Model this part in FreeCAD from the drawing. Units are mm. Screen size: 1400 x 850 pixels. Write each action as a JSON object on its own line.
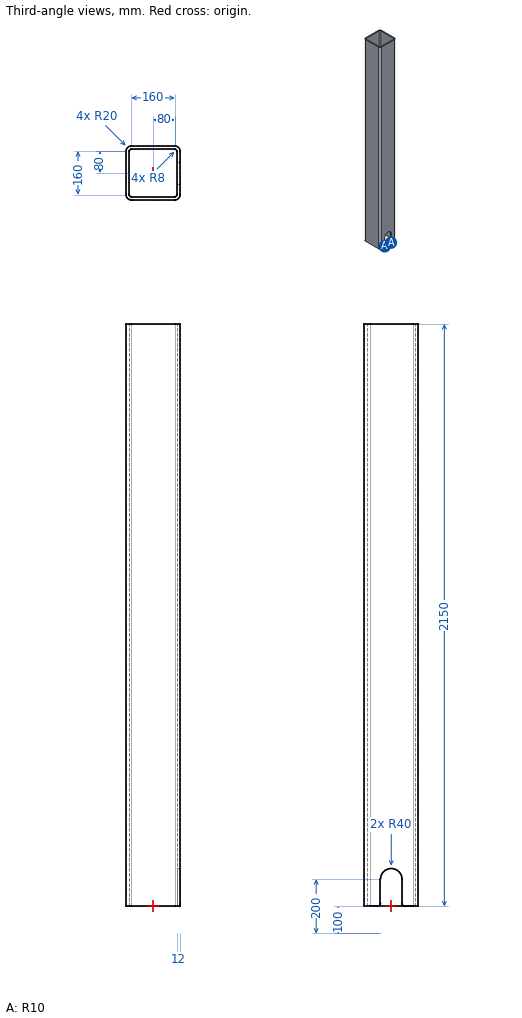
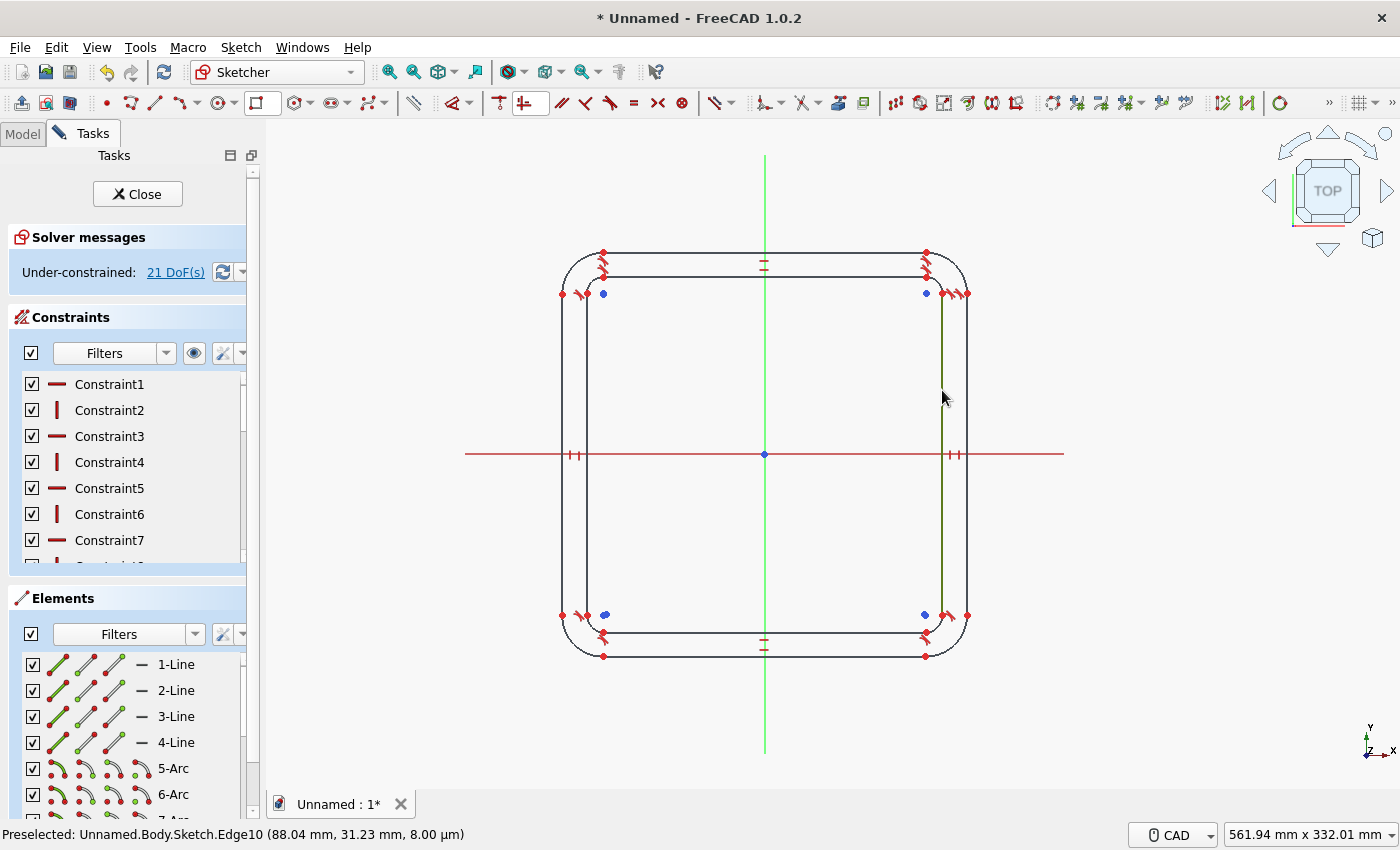
{"action": "left_click", "coordinate": [937, 627]}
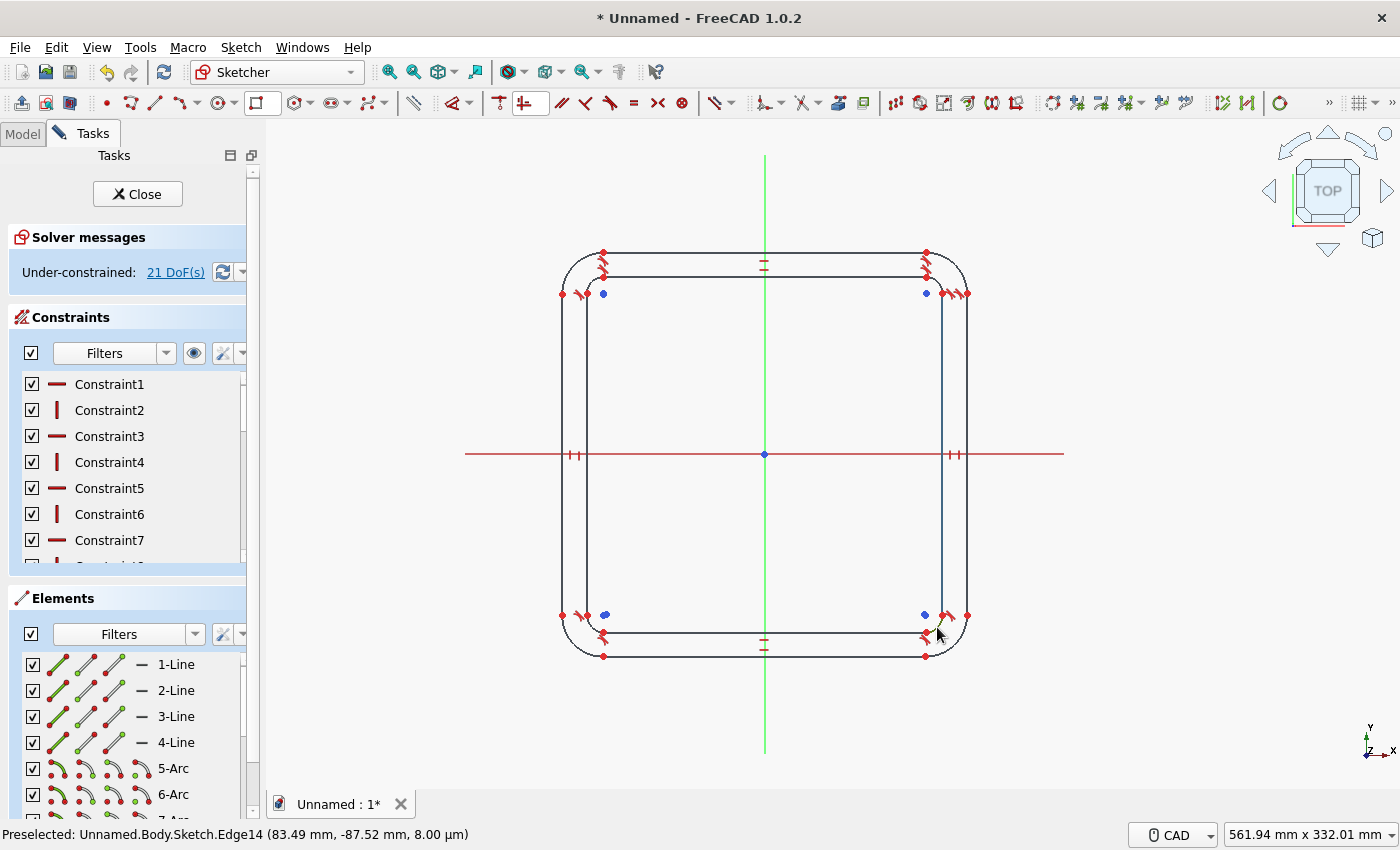
{"action": "left_click", "coordinate": [610, 104]}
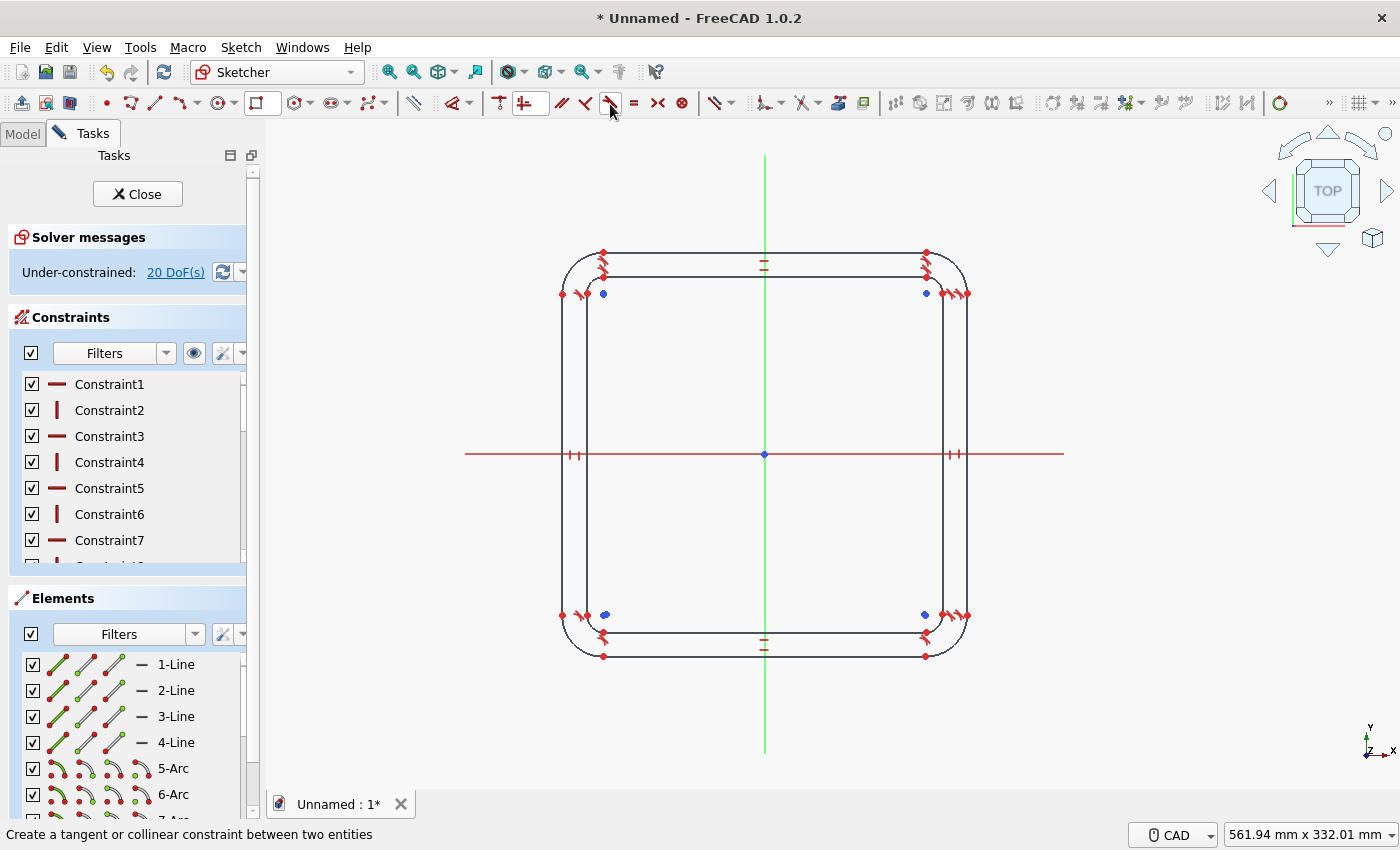
{"action": "left_click", "coordinate": [829, 633]}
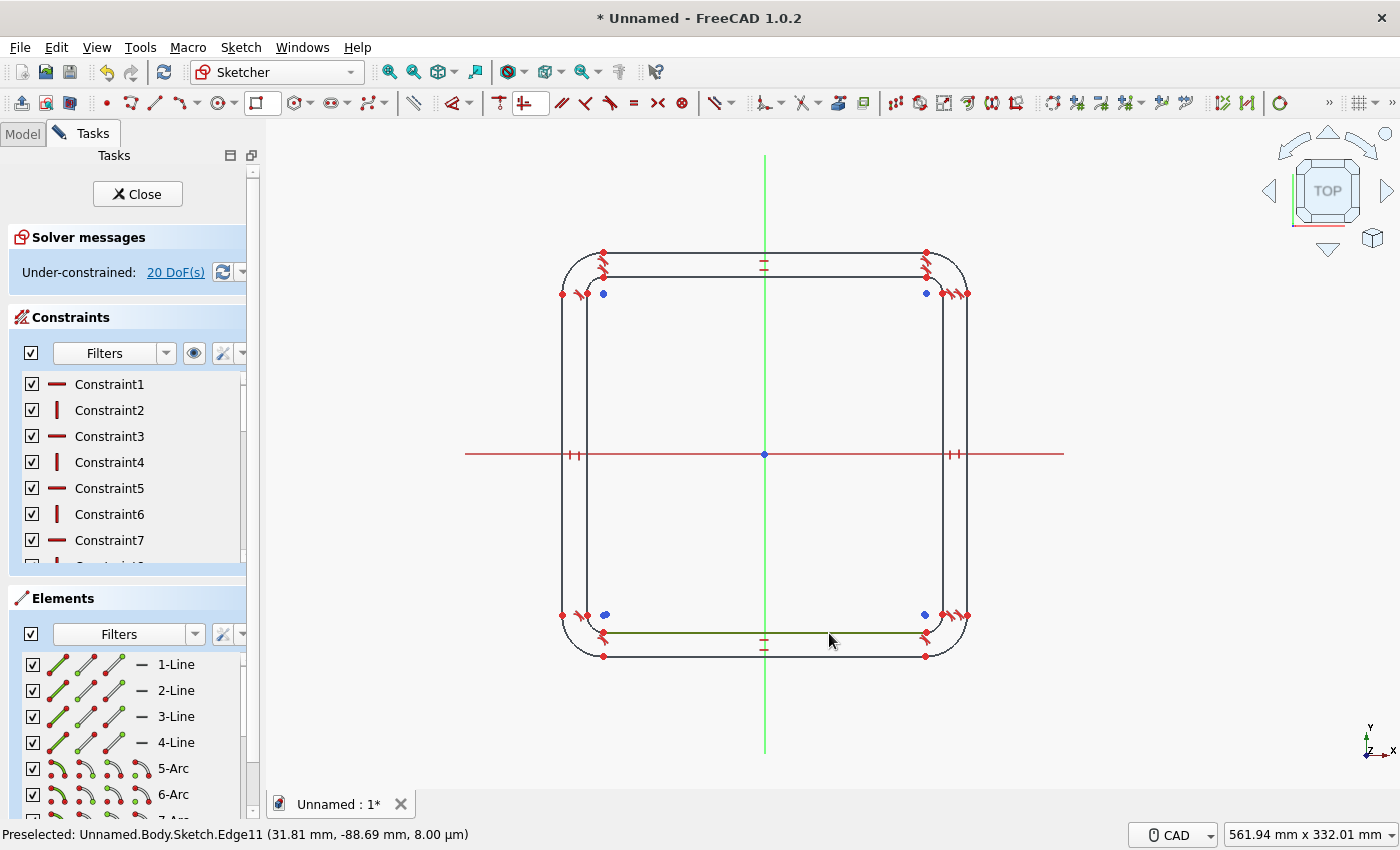
{"action": "left_click", "coordinate": [938, 627]}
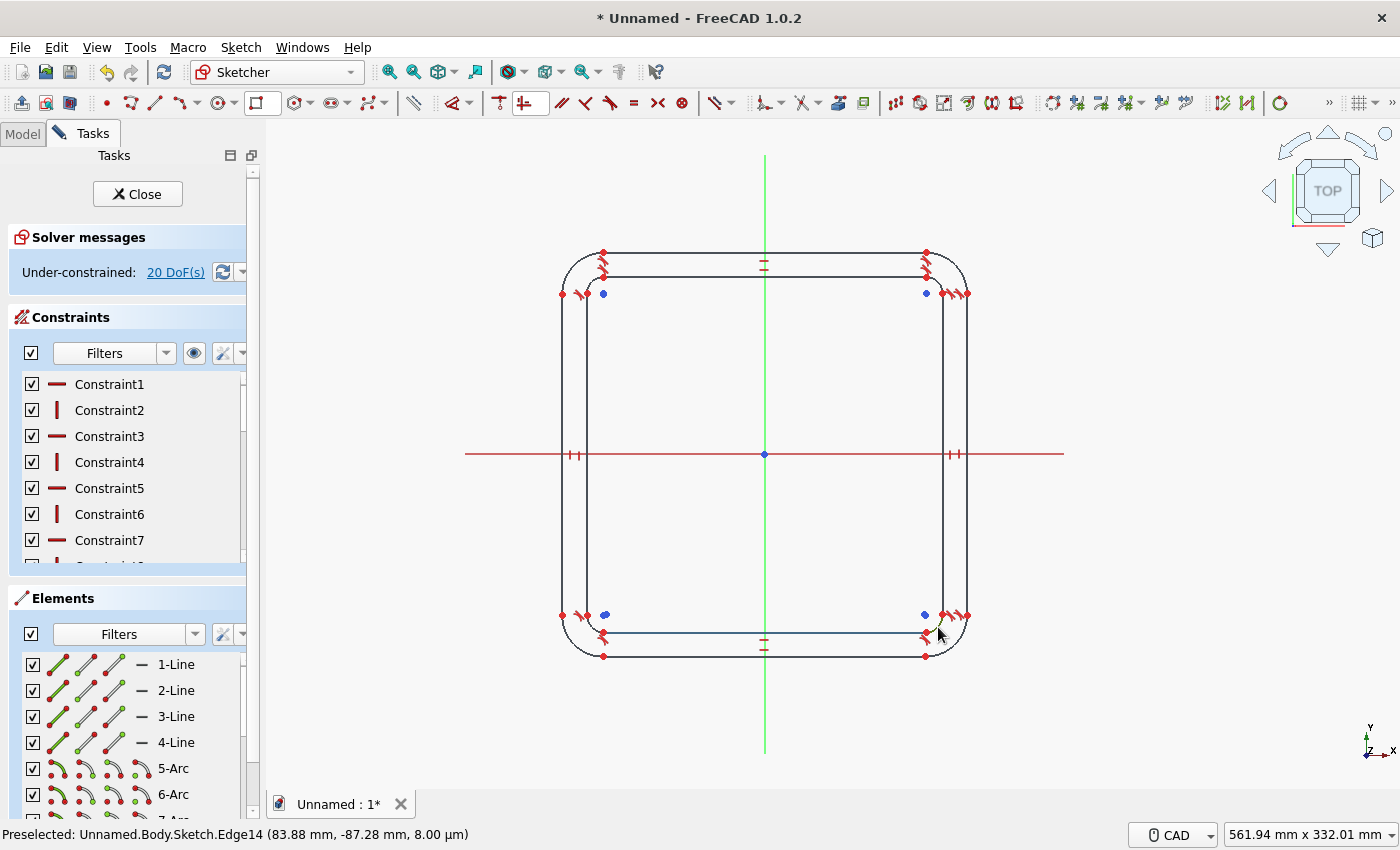
{"action": "left_click", "coordinate": [610, 104]}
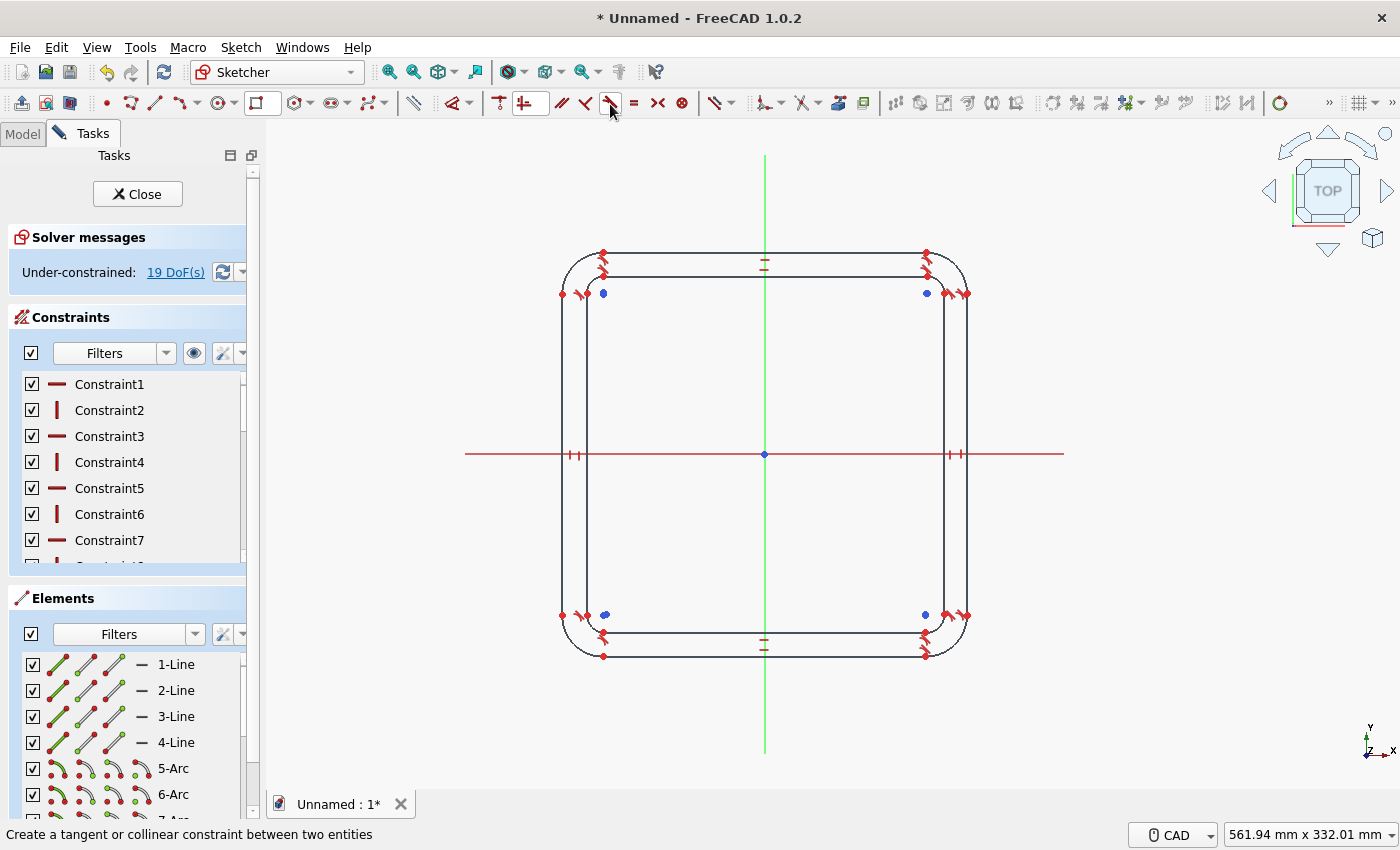
{"action": "left_click", "coordinate": [829, 633]}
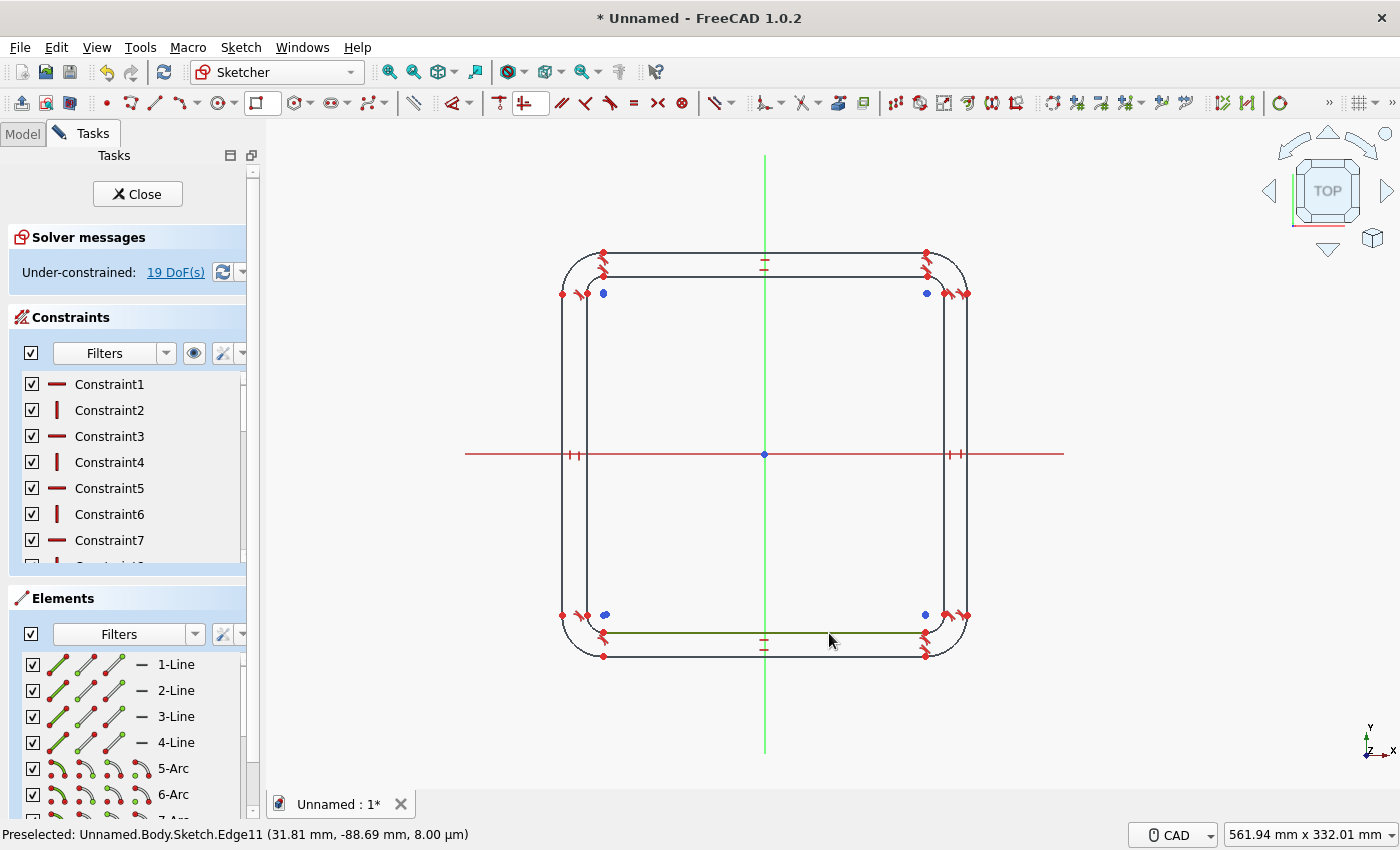
{"action": "left_click", "coordinate": [592, 627]}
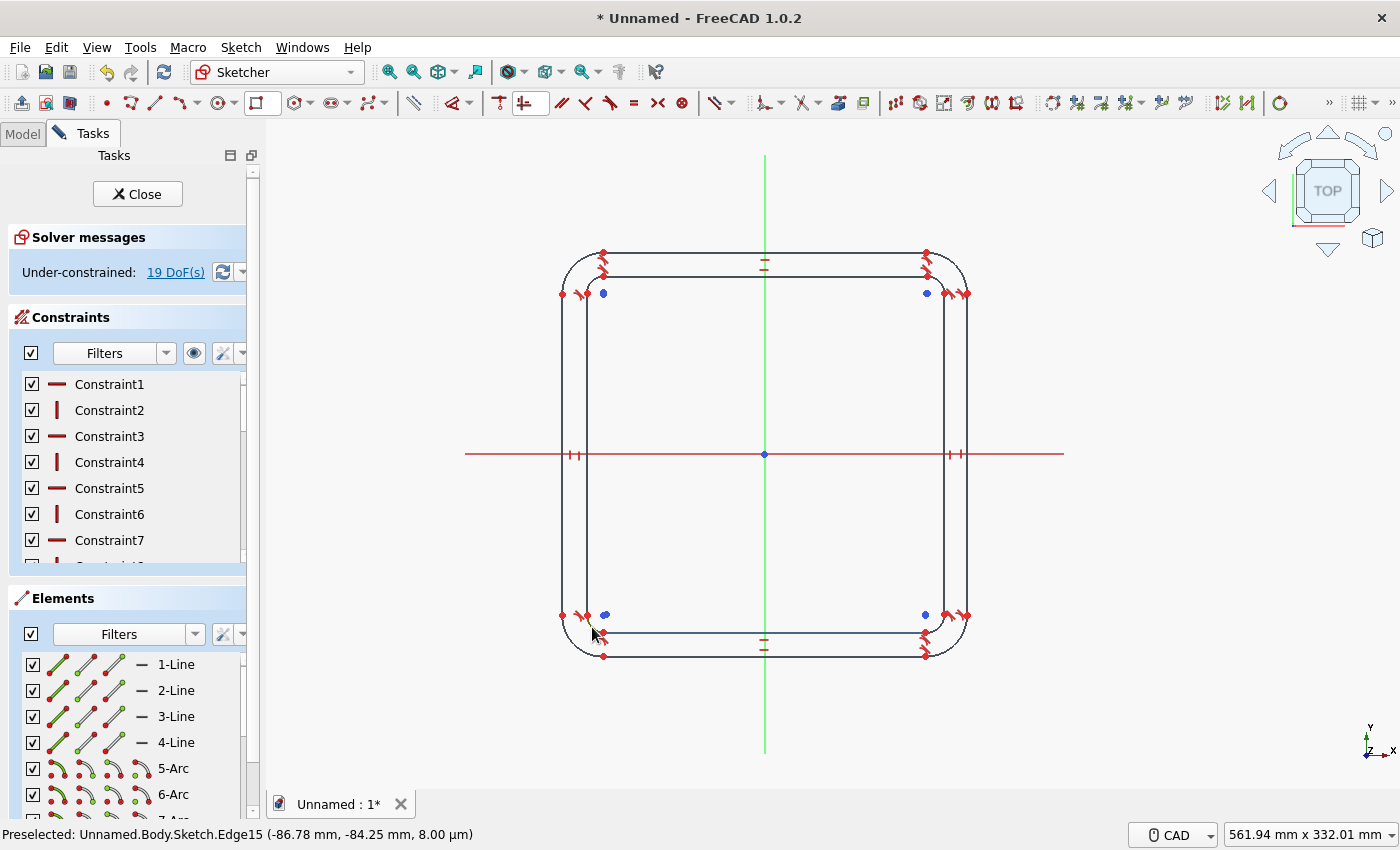
{"action": "left_click", "coordinate": [610, 104]}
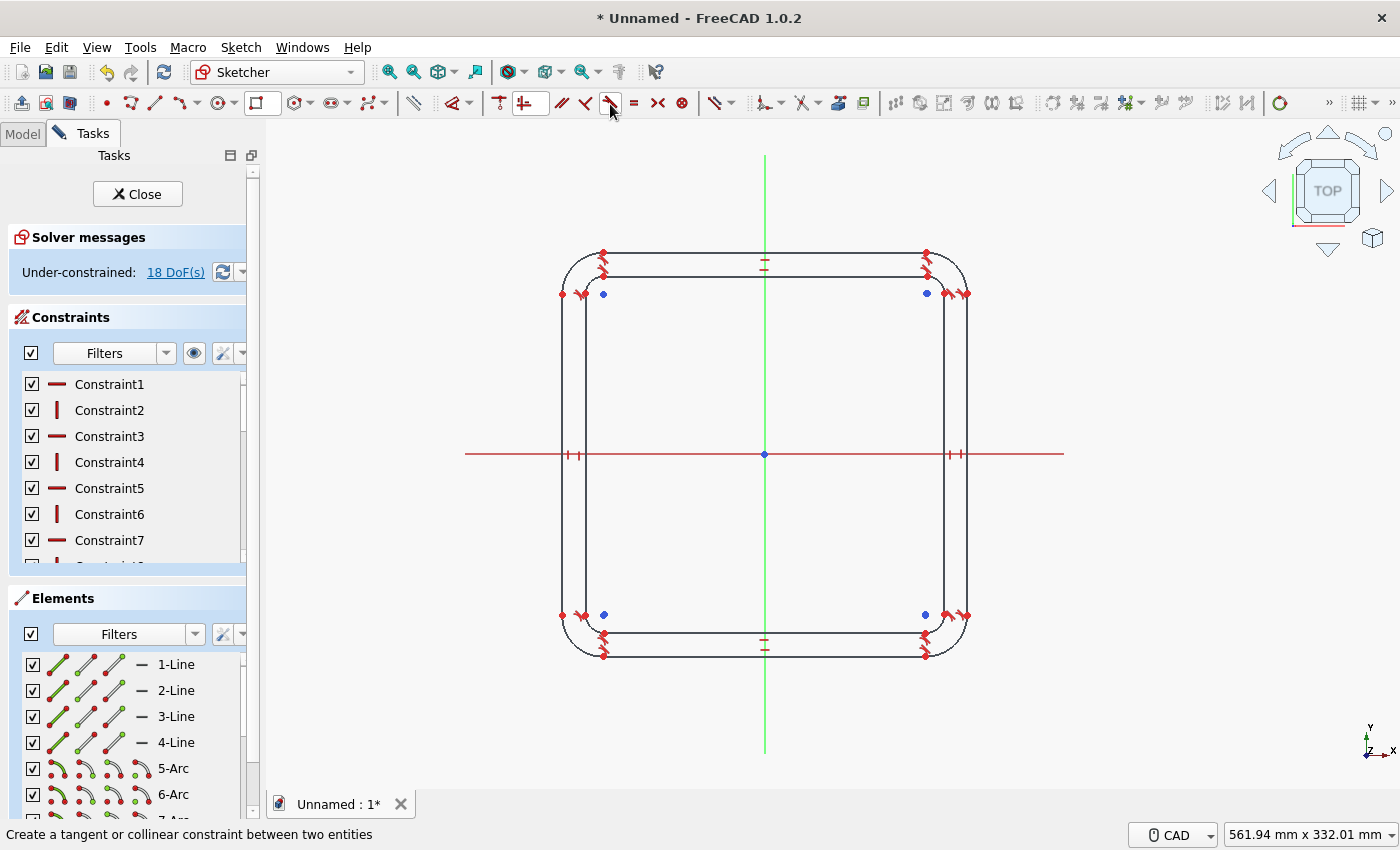
{"action": "left_click", "coordinate": [586, 519]}